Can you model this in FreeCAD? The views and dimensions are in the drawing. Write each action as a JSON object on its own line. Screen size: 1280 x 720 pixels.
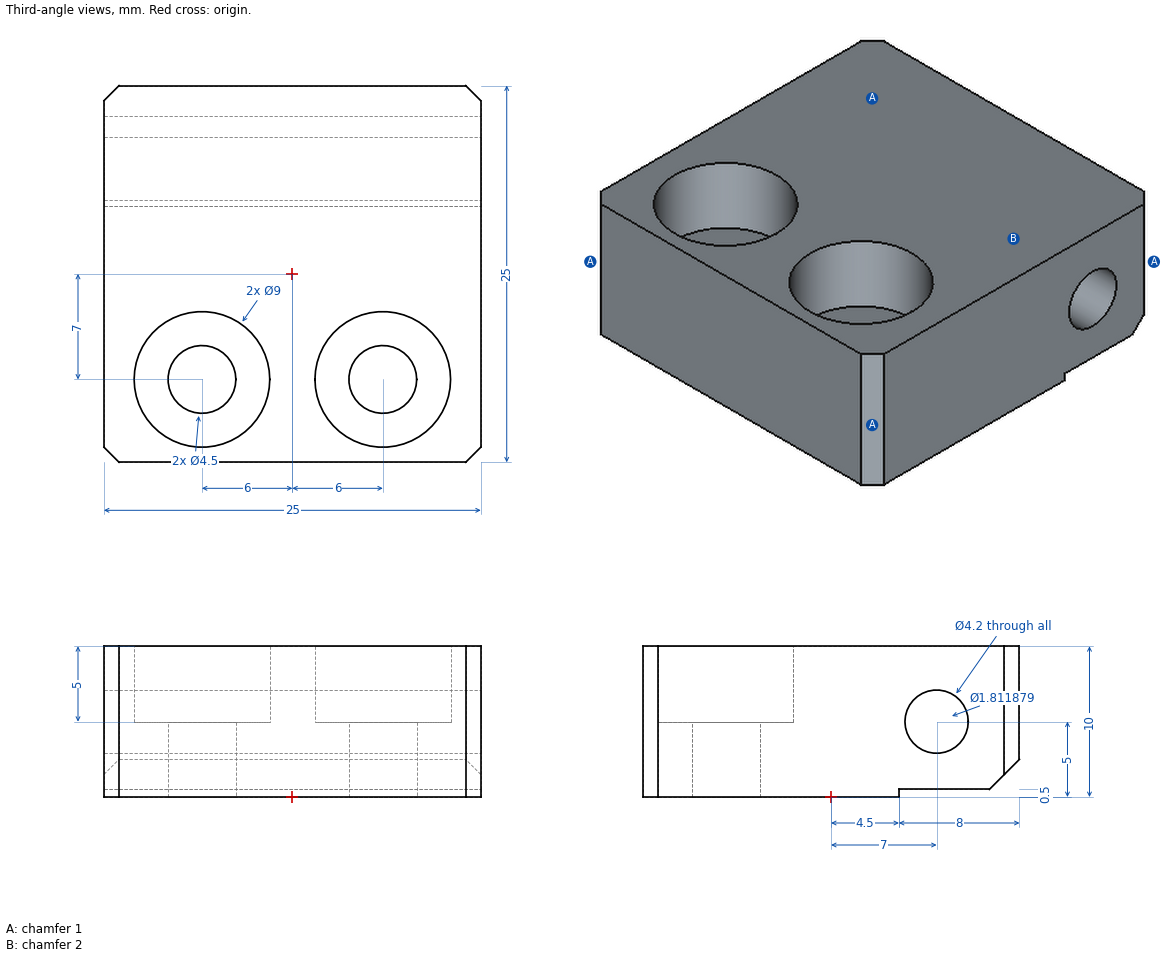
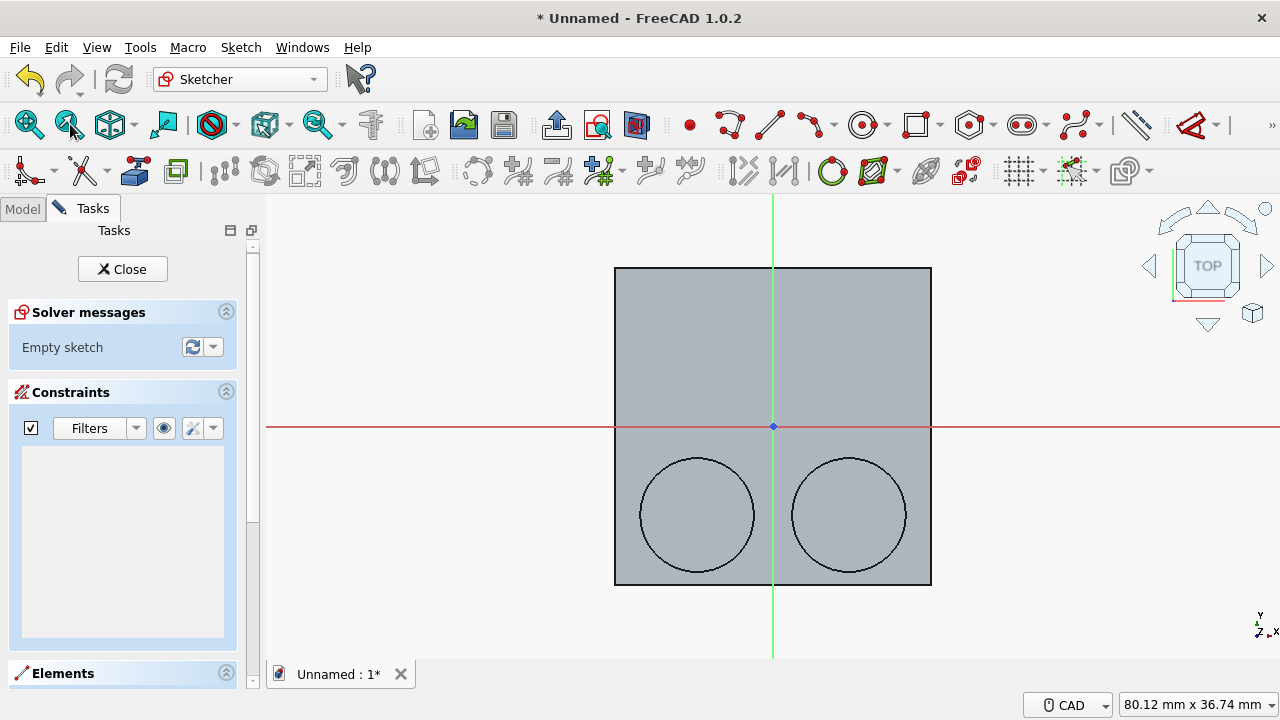
{"action": "scroll", "coordinate": [813, 519], "scroll_direction": "up", "scroll_amount": 5}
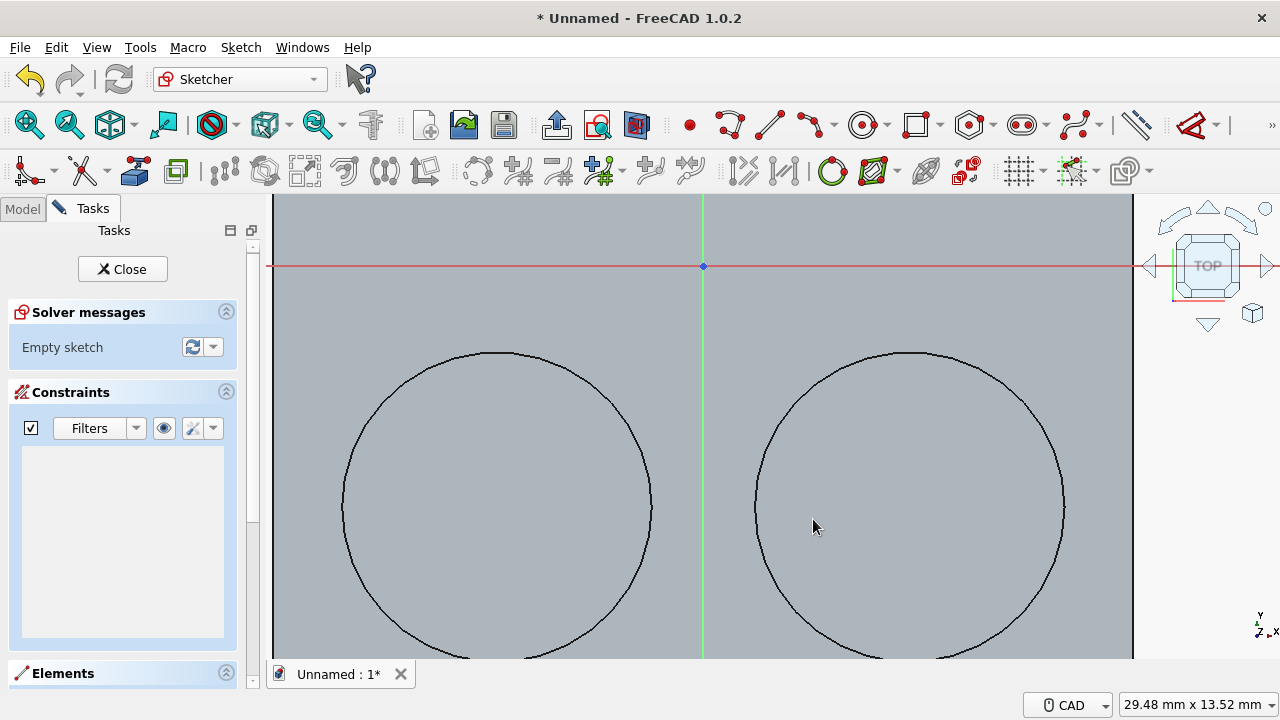
{"action": "key", "text": "g c"}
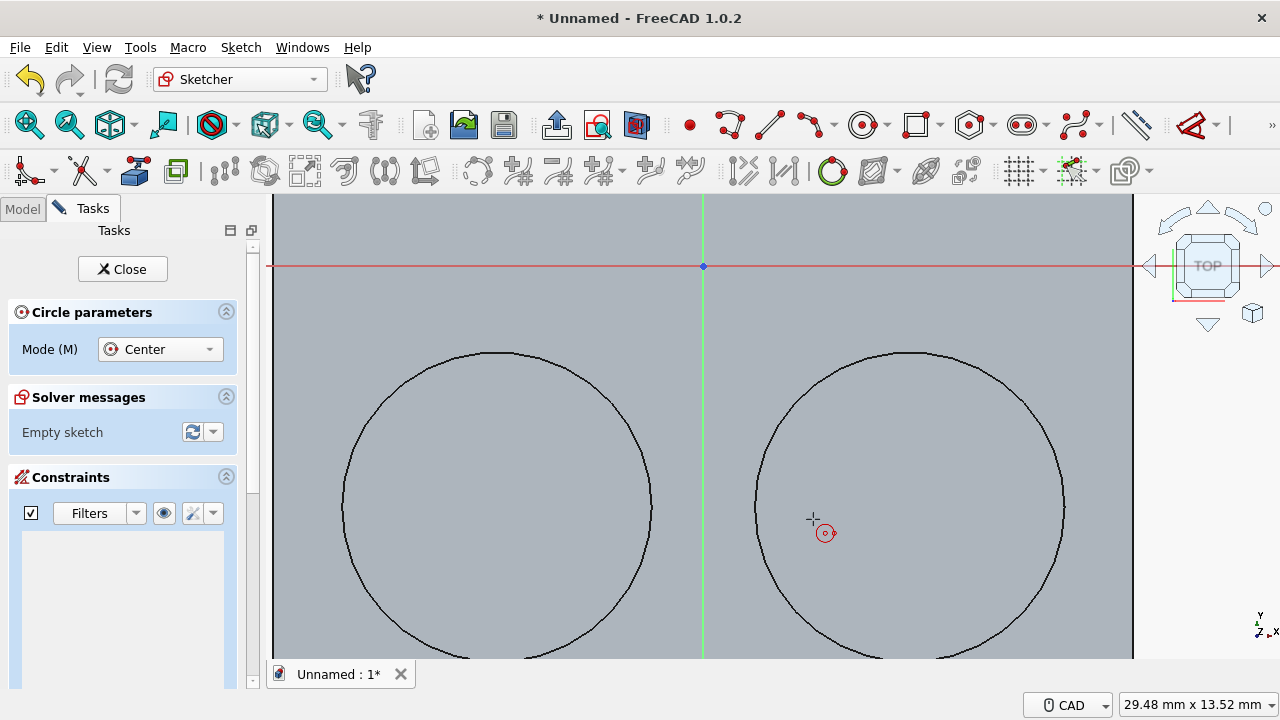
{"action": "left_click", "coordinate": [497, 507]}
{"action": "left_click", "coordinate": [552, 452]}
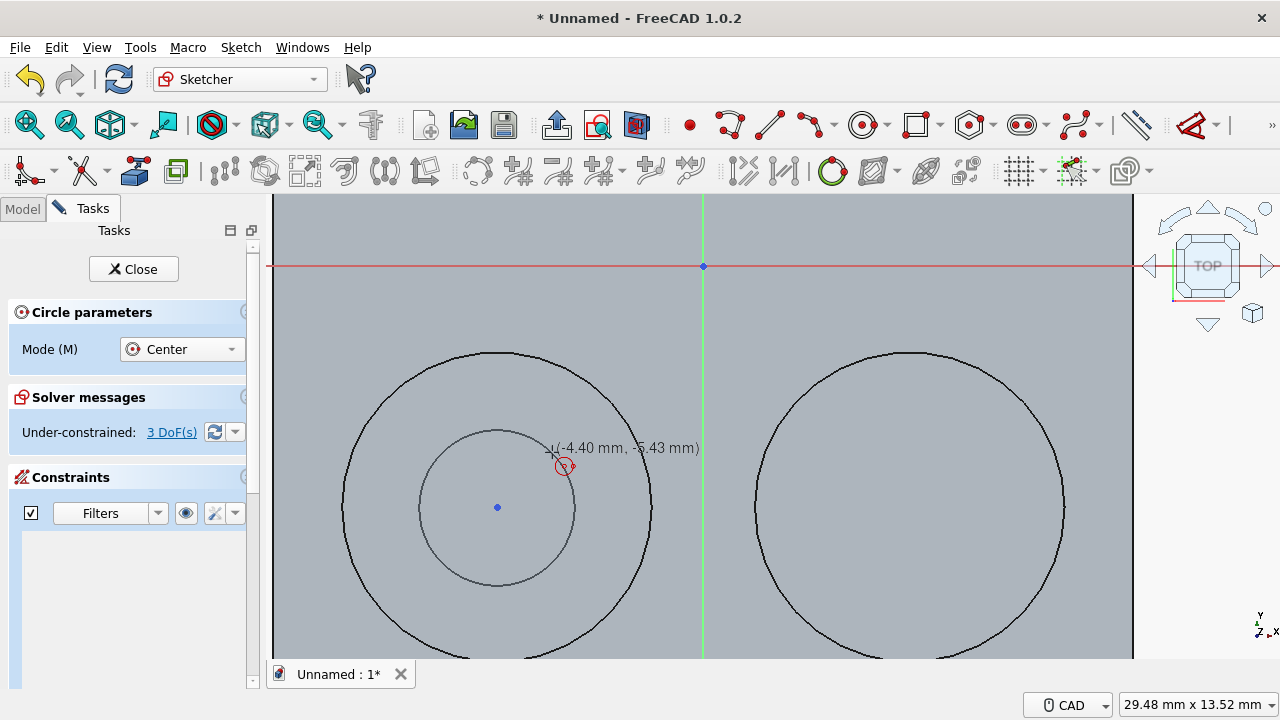
{"action": "left_click", "coordinate": [910, 507]}
{"action": "left_click", "coordinate": [964, 452]}
{"action": "key", "text": "Escape"}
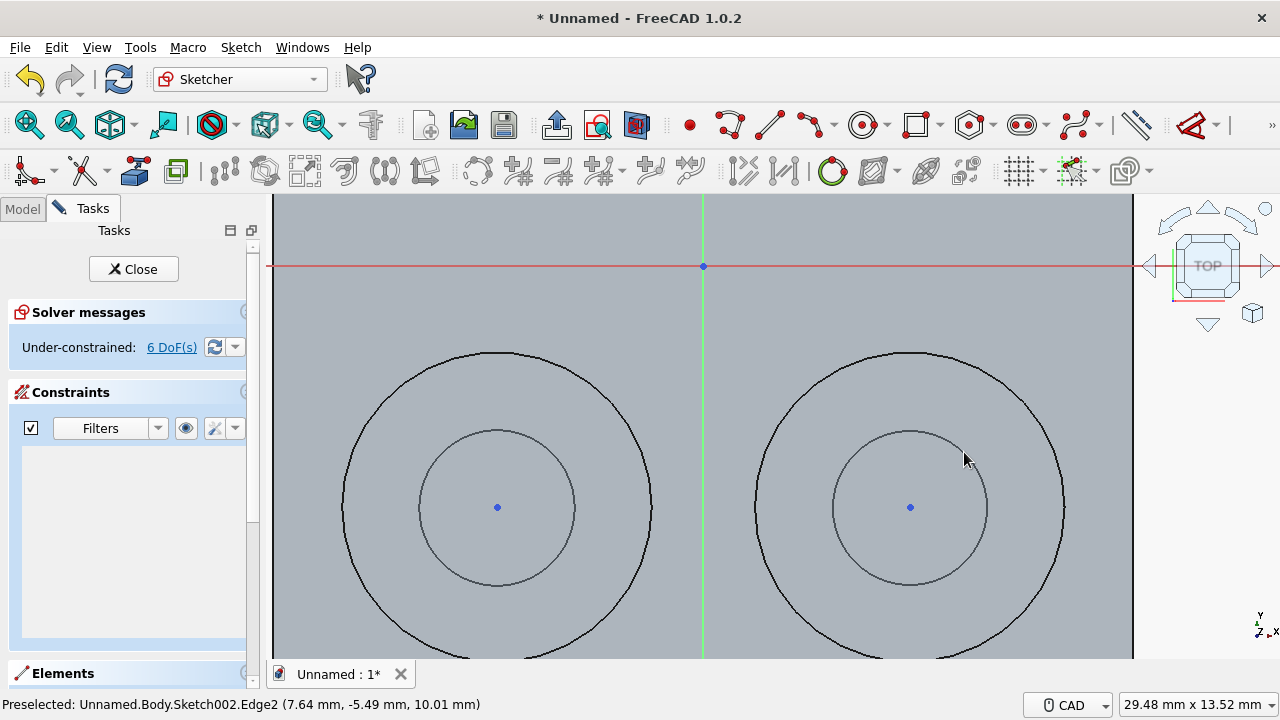
{"action": "left_click", "coordinate": [552, 453]}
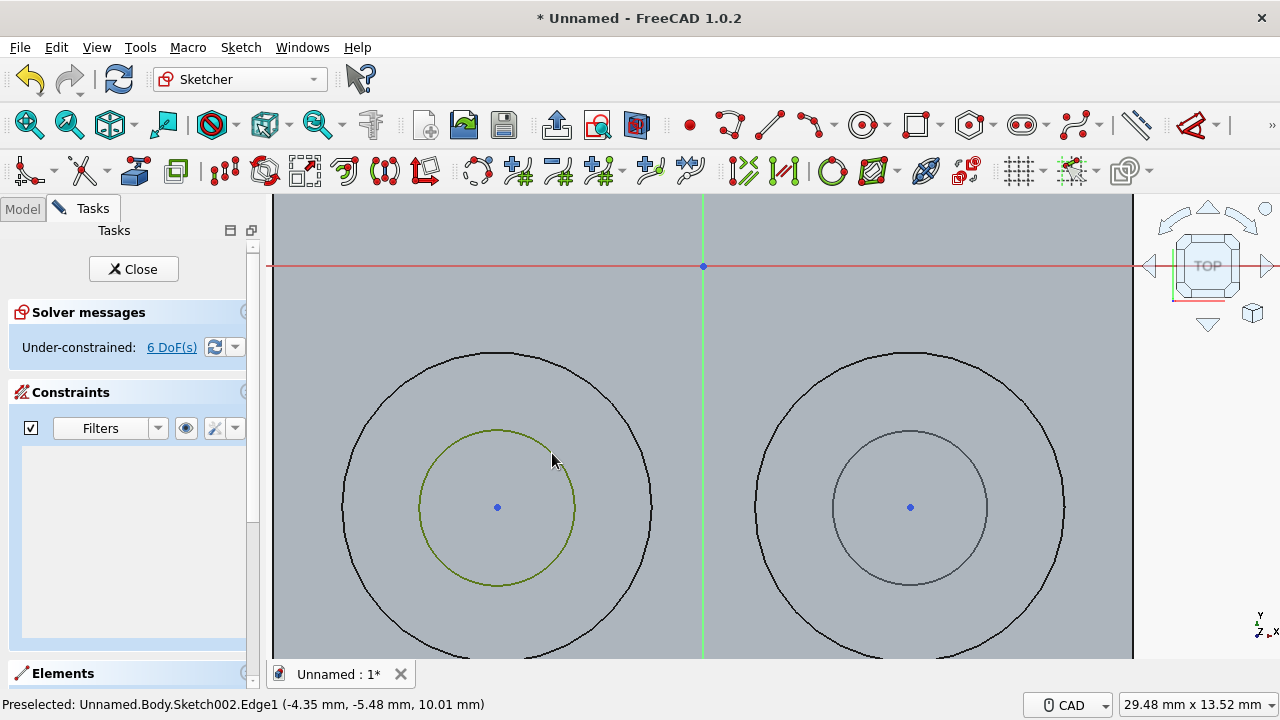
{"action": "left_click", "coordinate": [964, 453]}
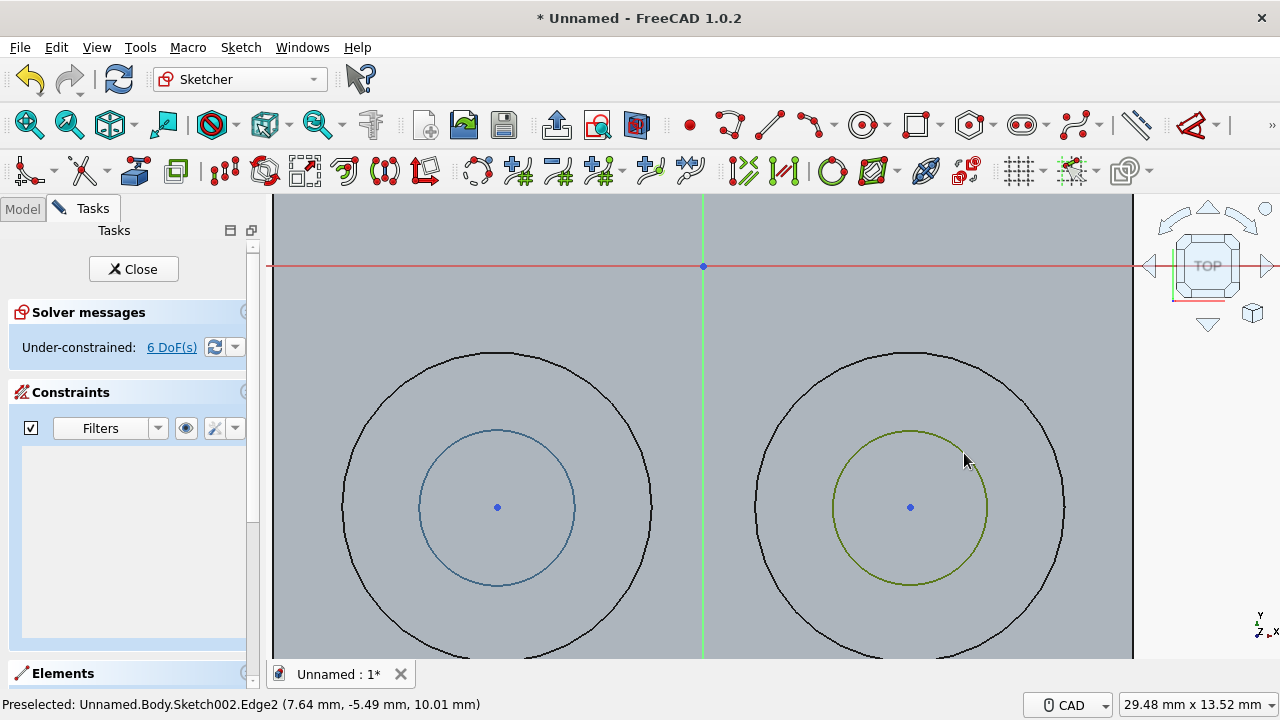
{"action": "key", "text": "e"}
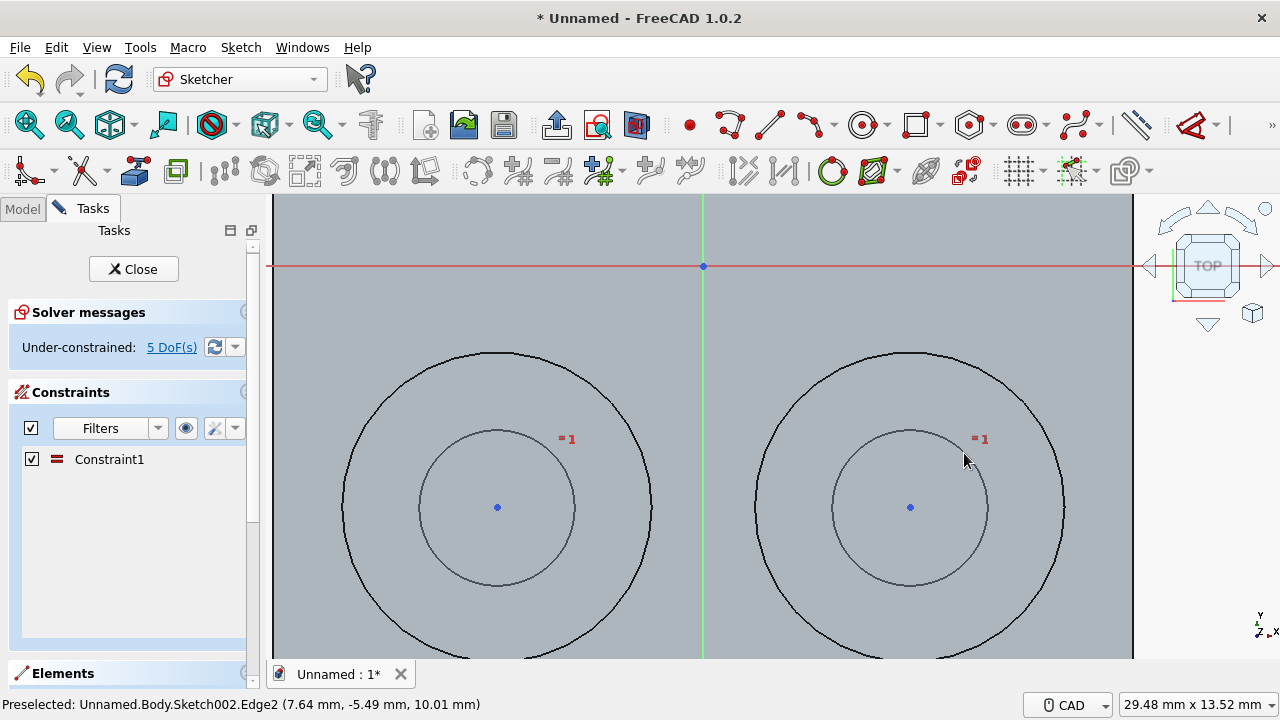
{"action": "left_click", "coordinate": [497, 508]}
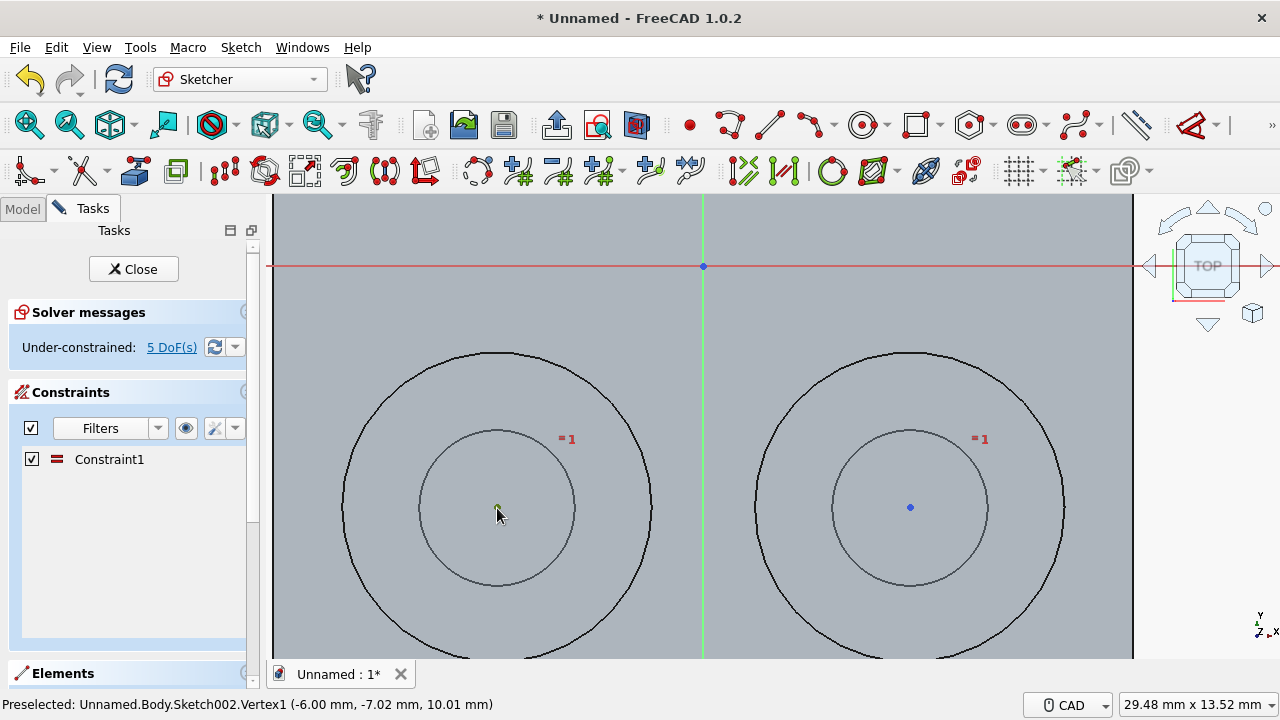
{"action": "left_click", "coordinate": [910, 508]}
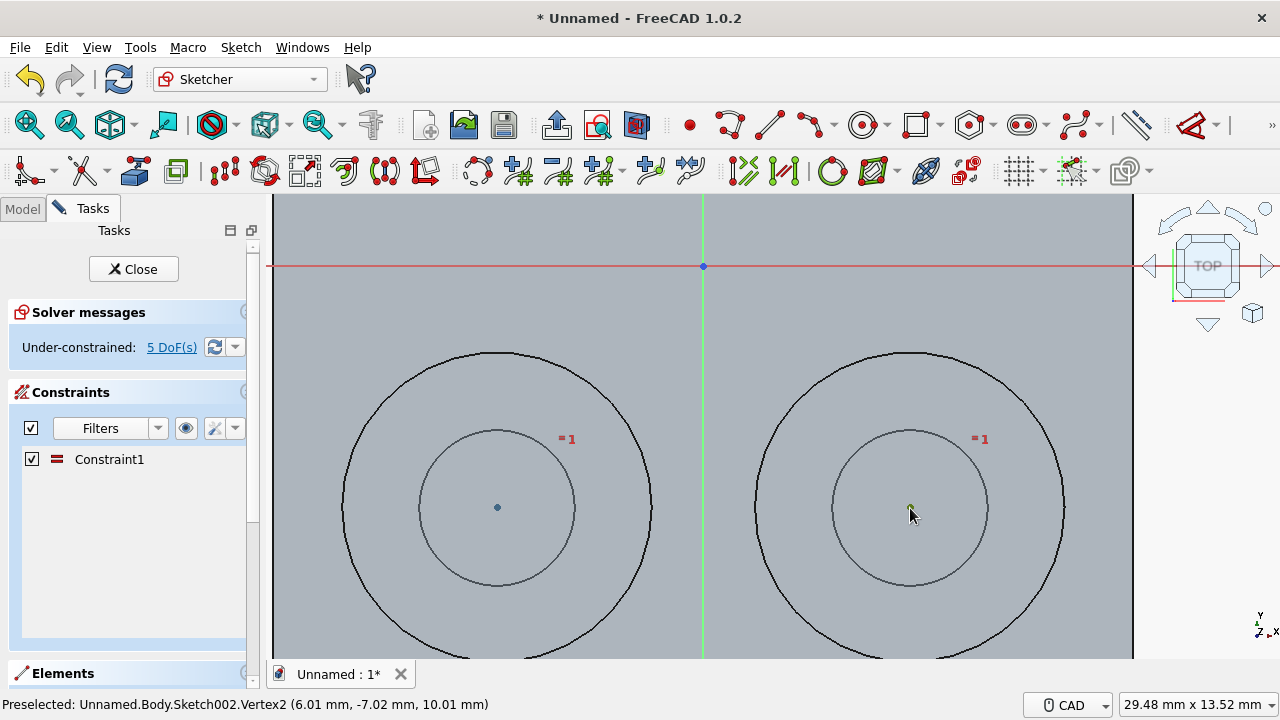
{"action": "key", "text": "h"}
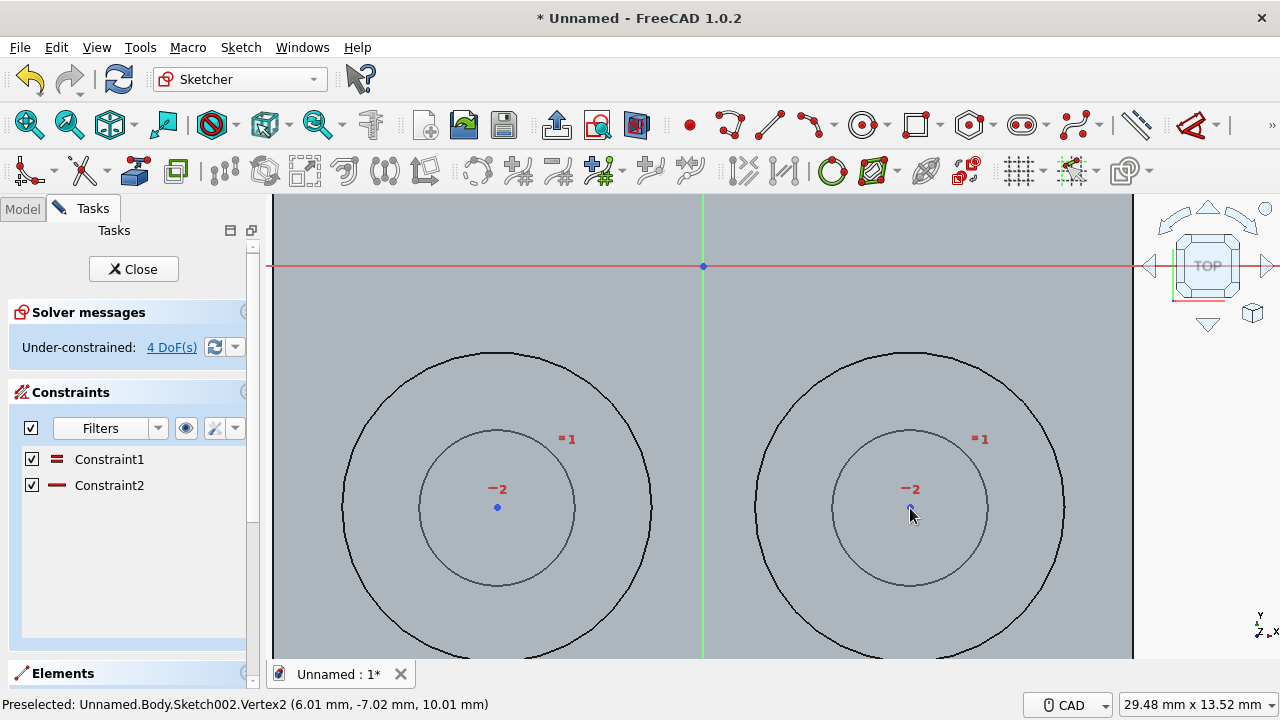
{"action": "key", "text": "d"}